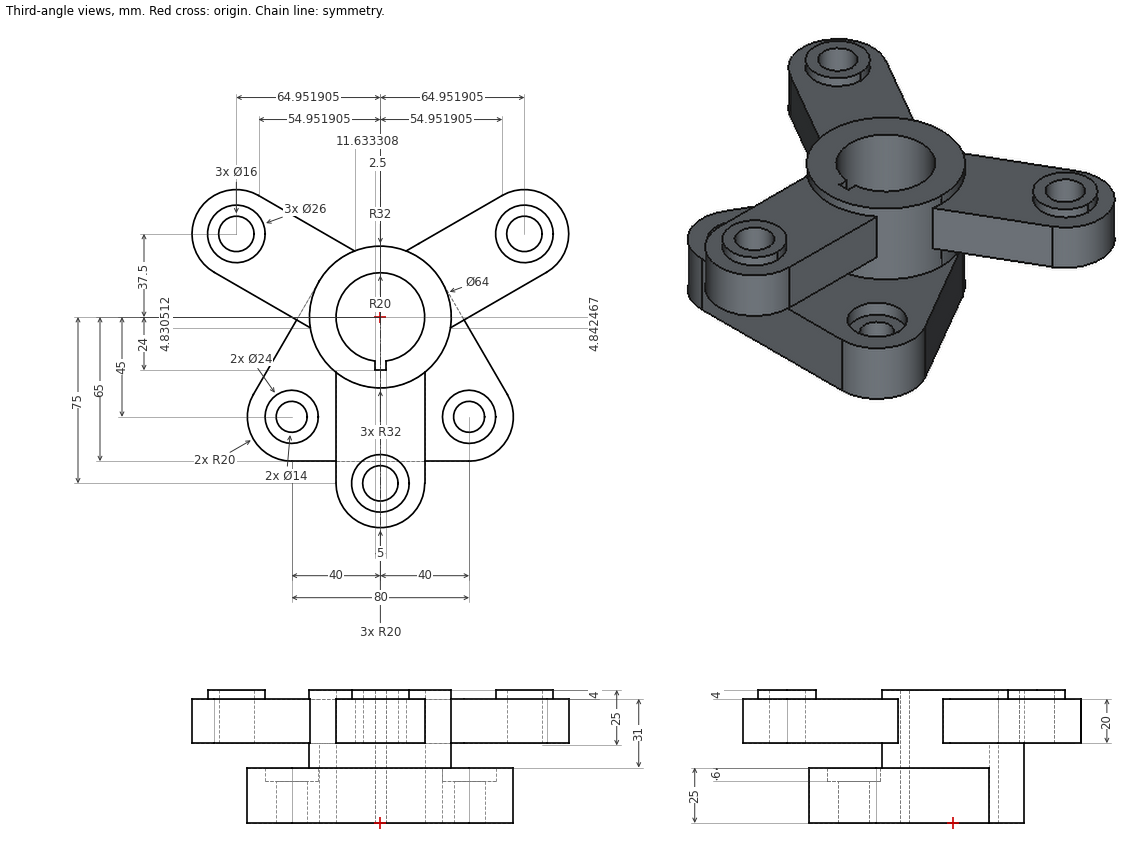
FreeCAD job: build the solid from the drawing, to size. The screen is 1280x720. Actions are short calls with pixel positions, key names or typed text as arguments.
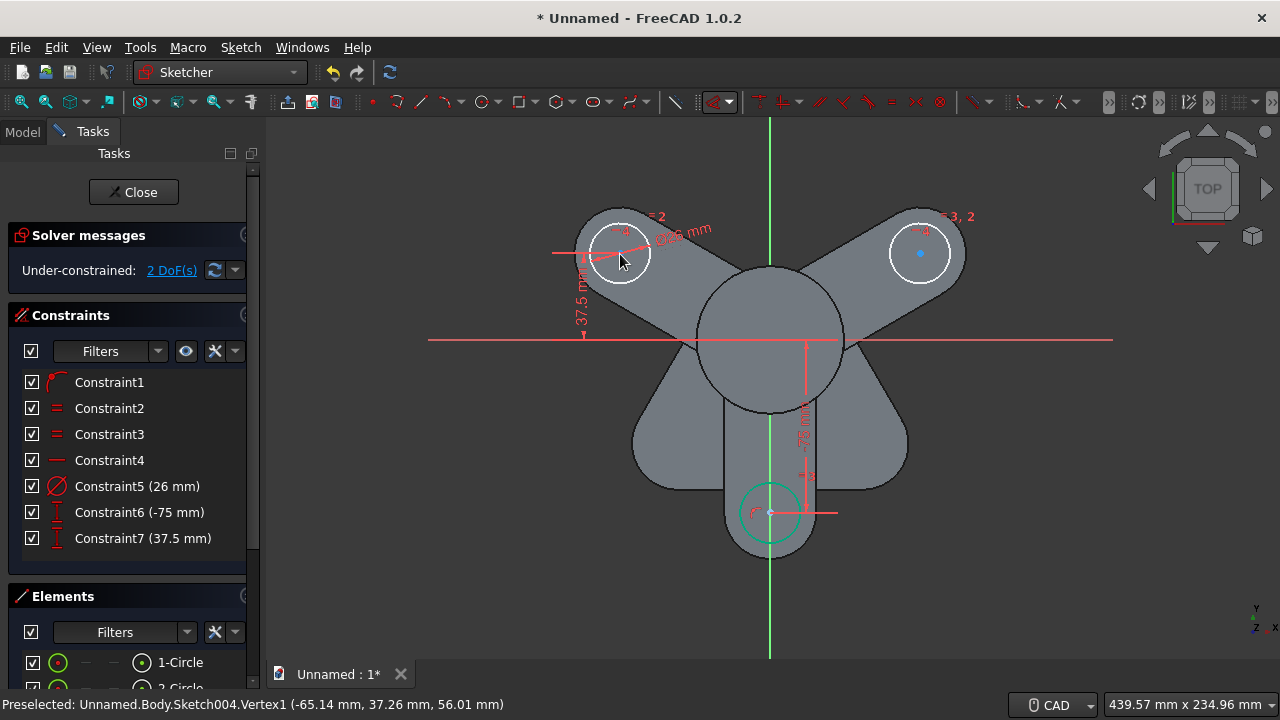
click(620, 253)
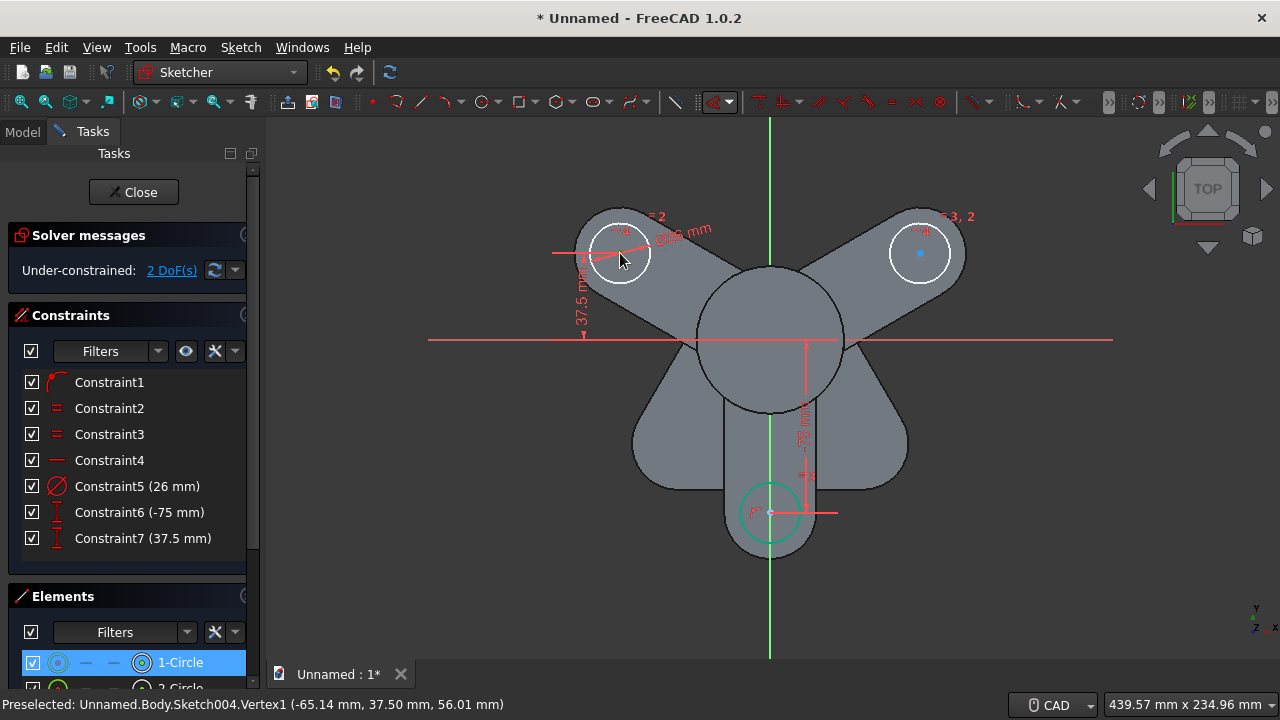
key(l)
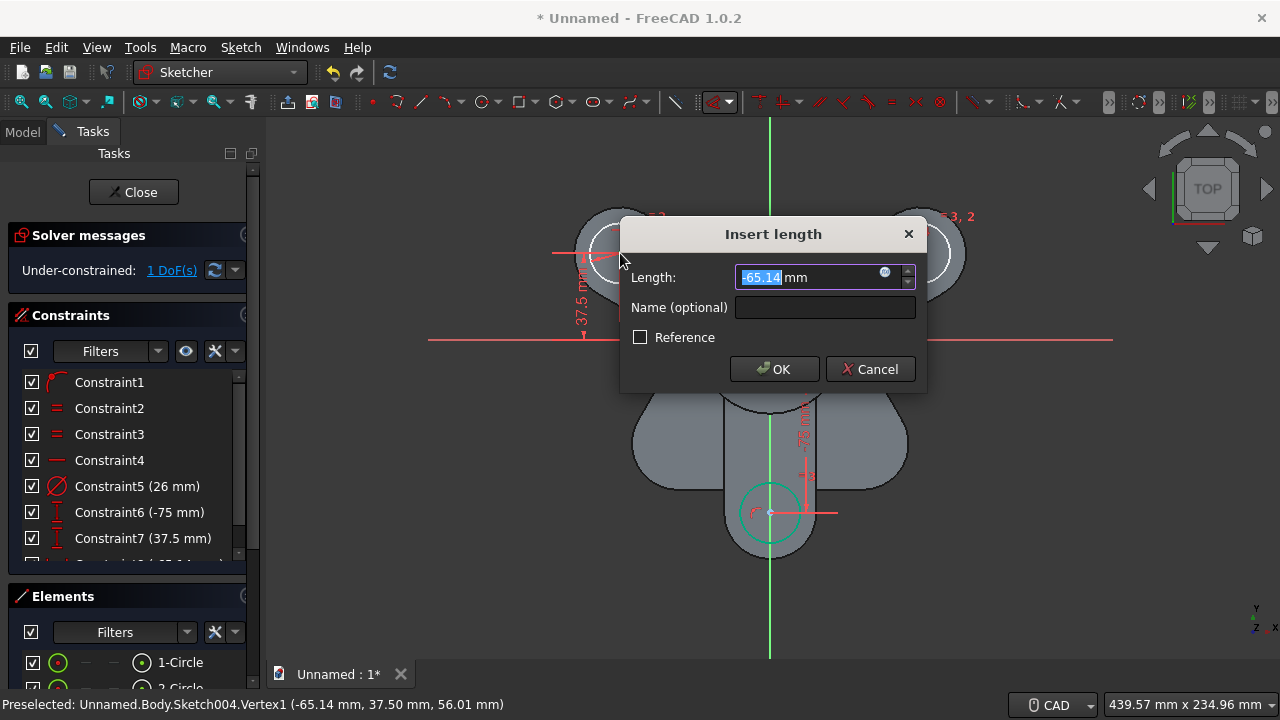
text(-64.951905)
key(Return)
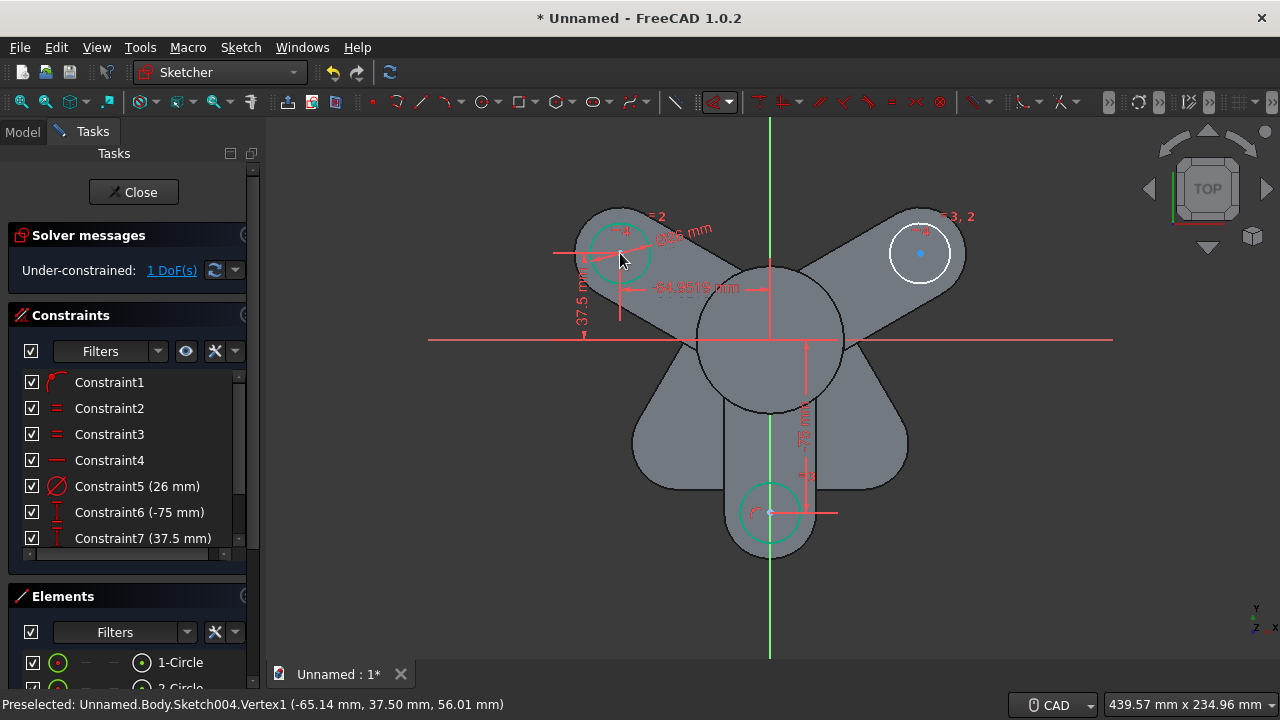
click(920, 253)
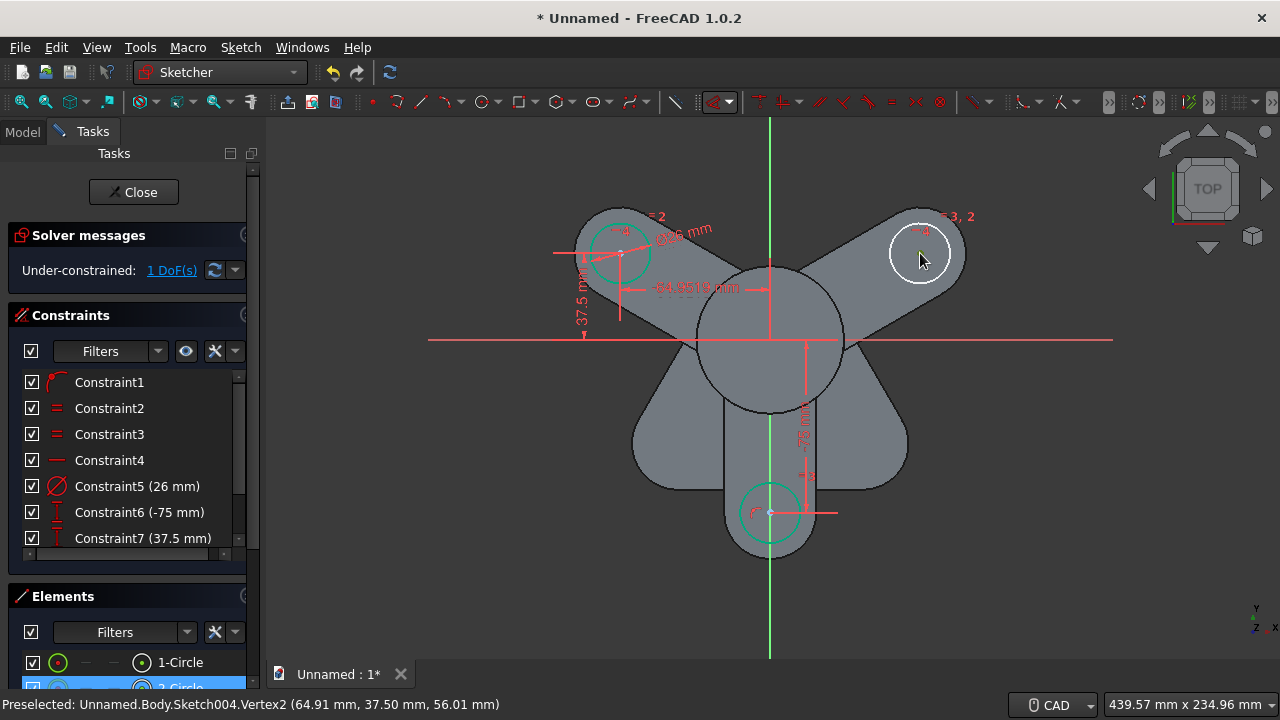
key(l)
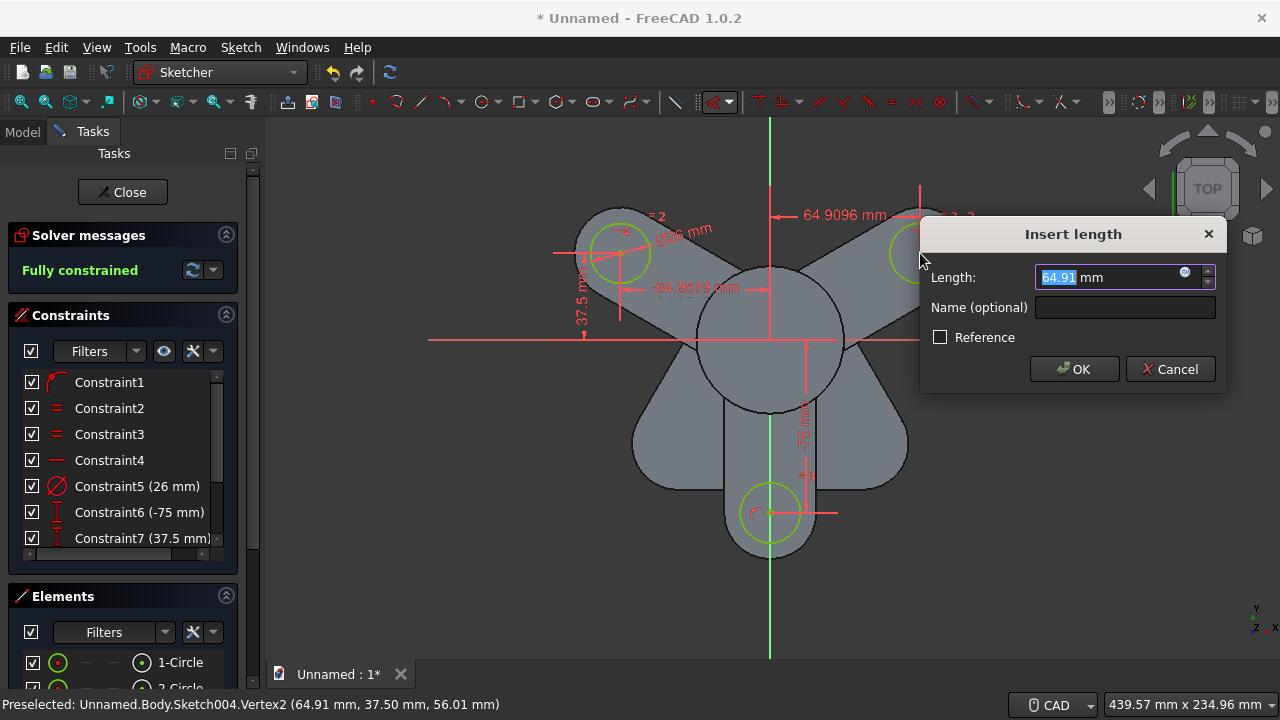
text(64.951905)
key(Return)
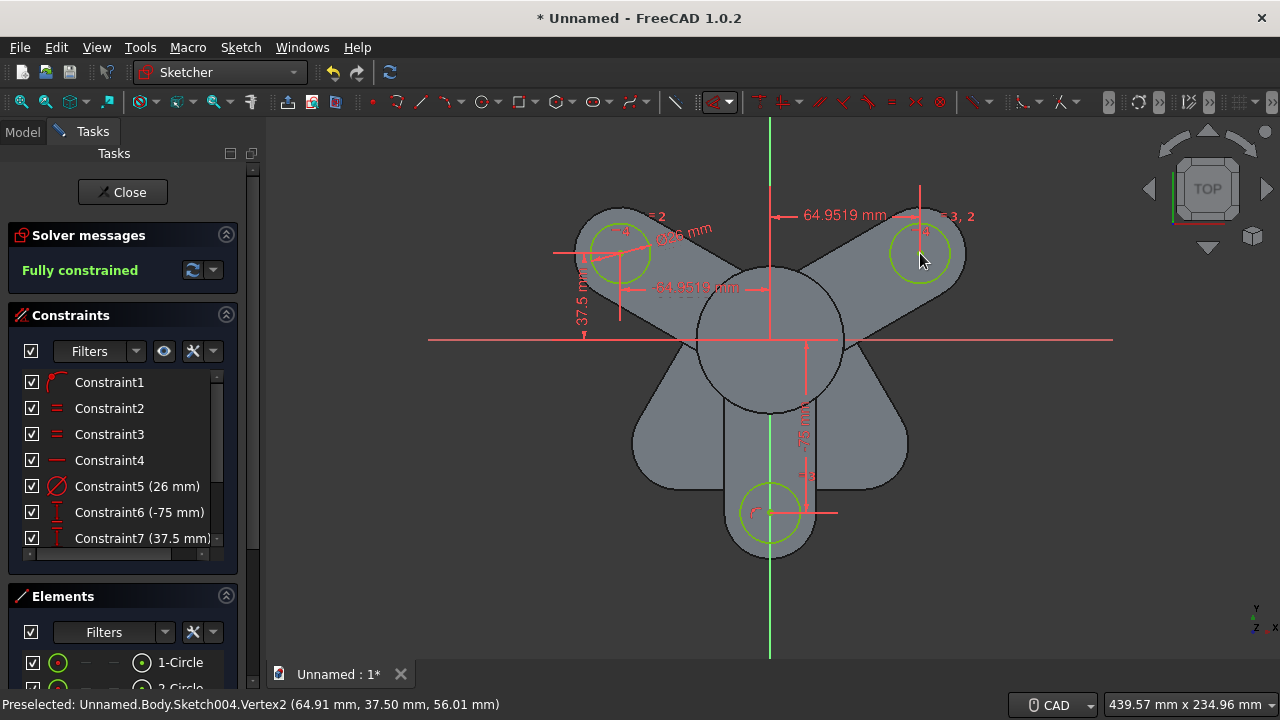
click(123, 192)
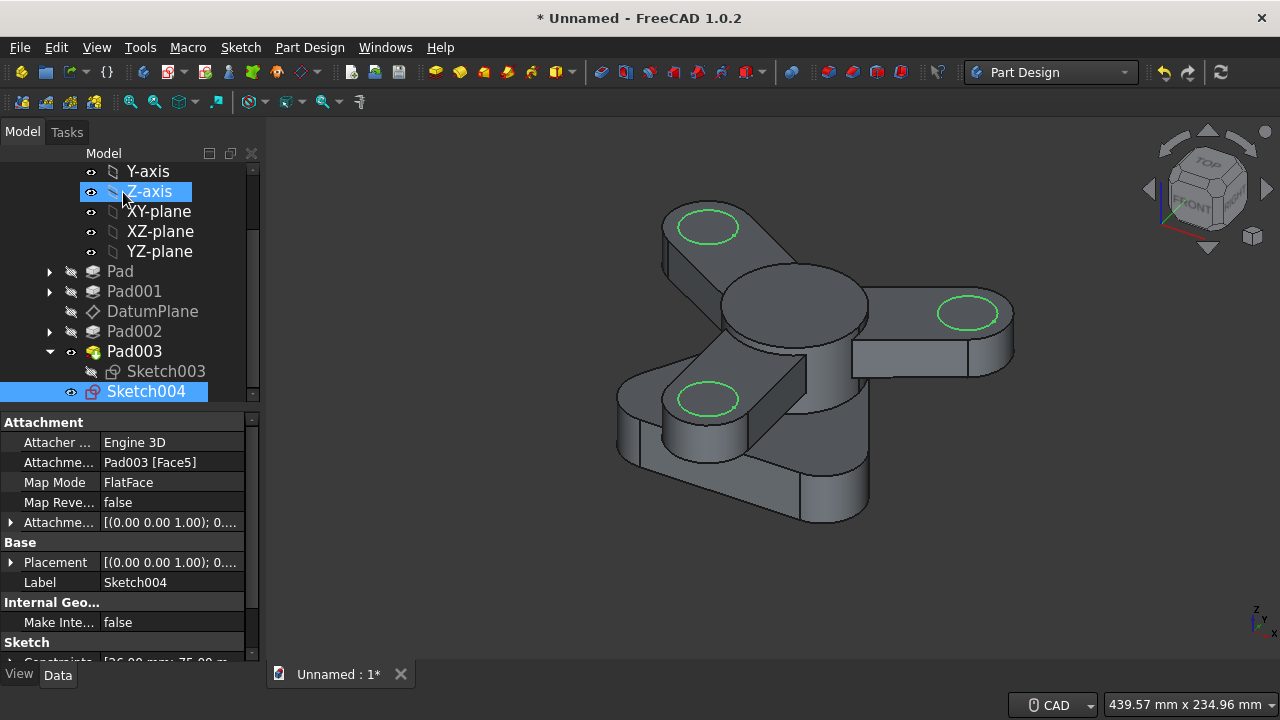
click(436, 72)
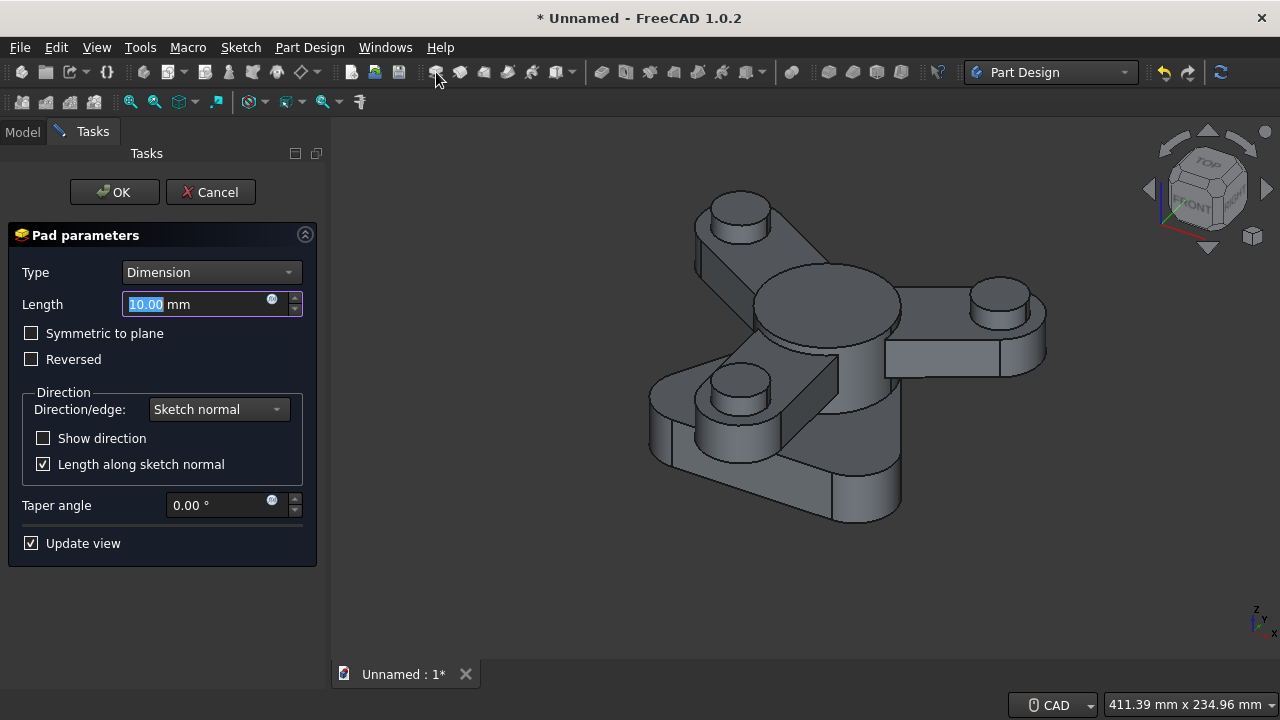
text(4)
key(Tab)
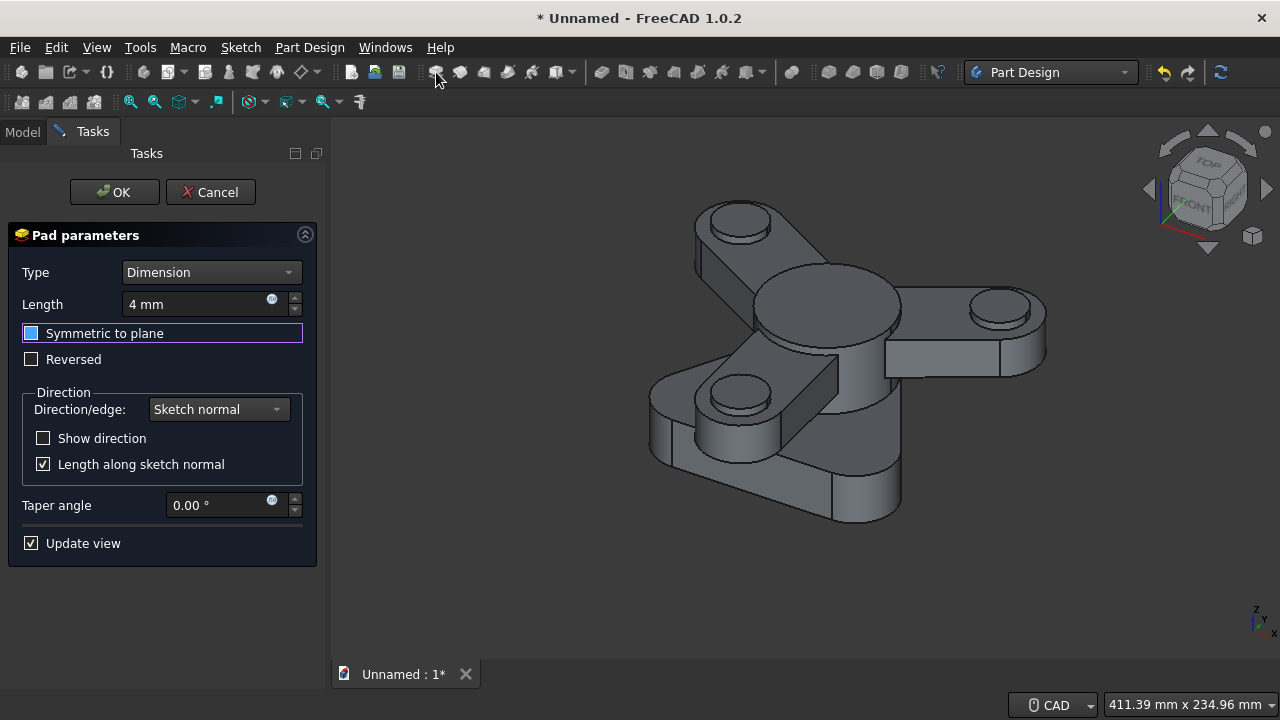
click(115, 192)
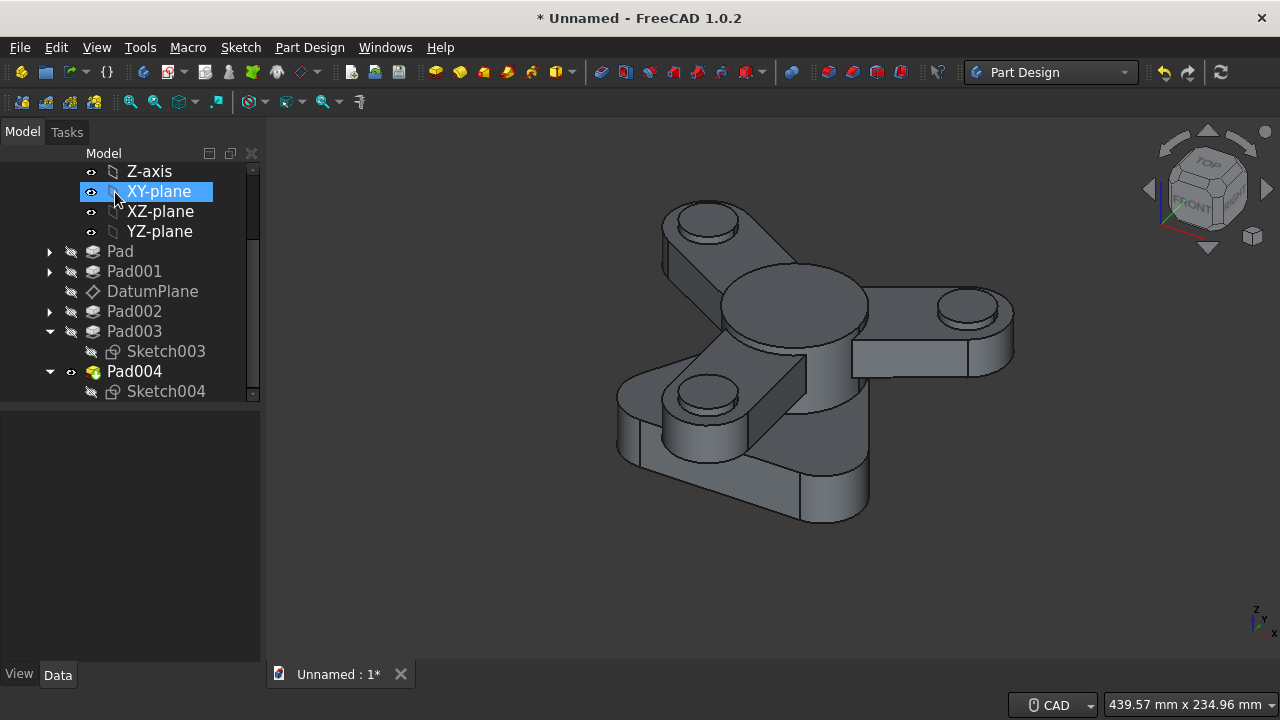
click(795, 305)